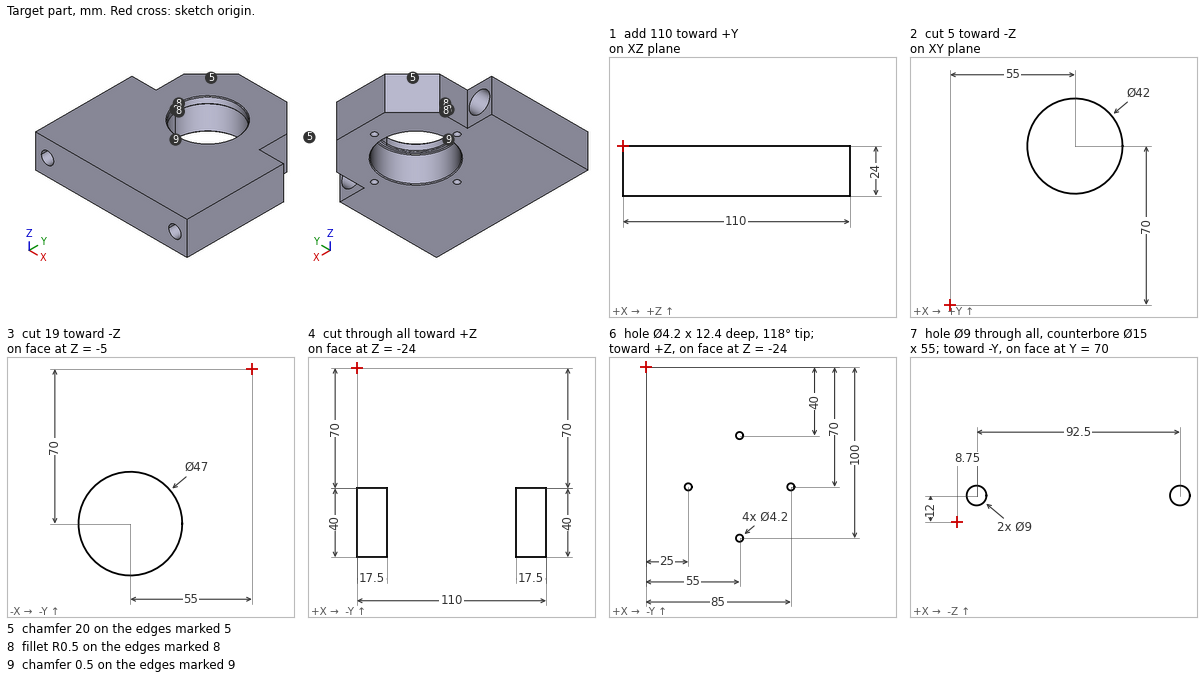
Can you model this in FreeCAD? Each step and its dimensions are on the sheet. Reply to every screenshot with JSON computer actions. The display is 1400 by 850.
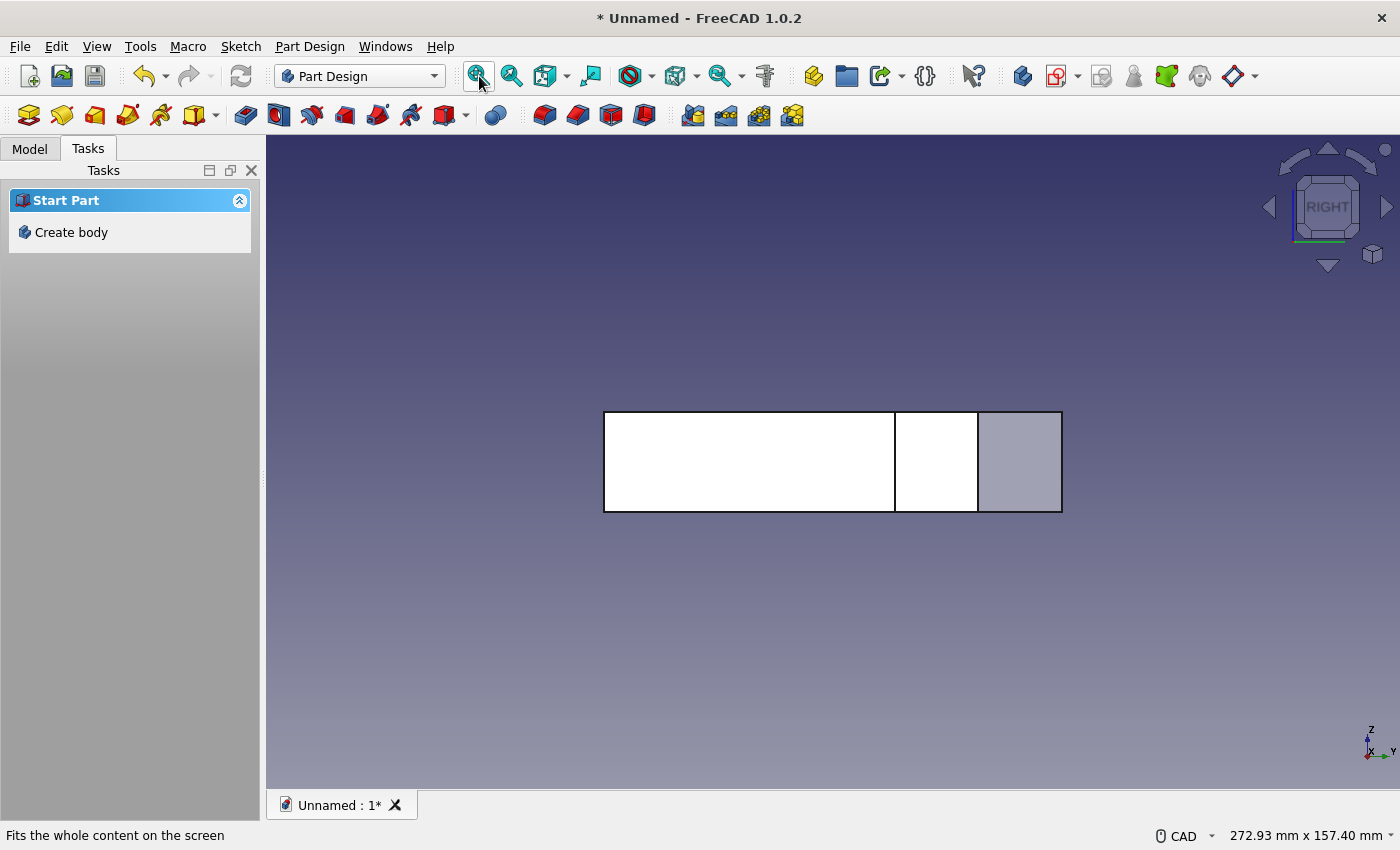
{"action": "left_click", "coordinate": [479, 76]}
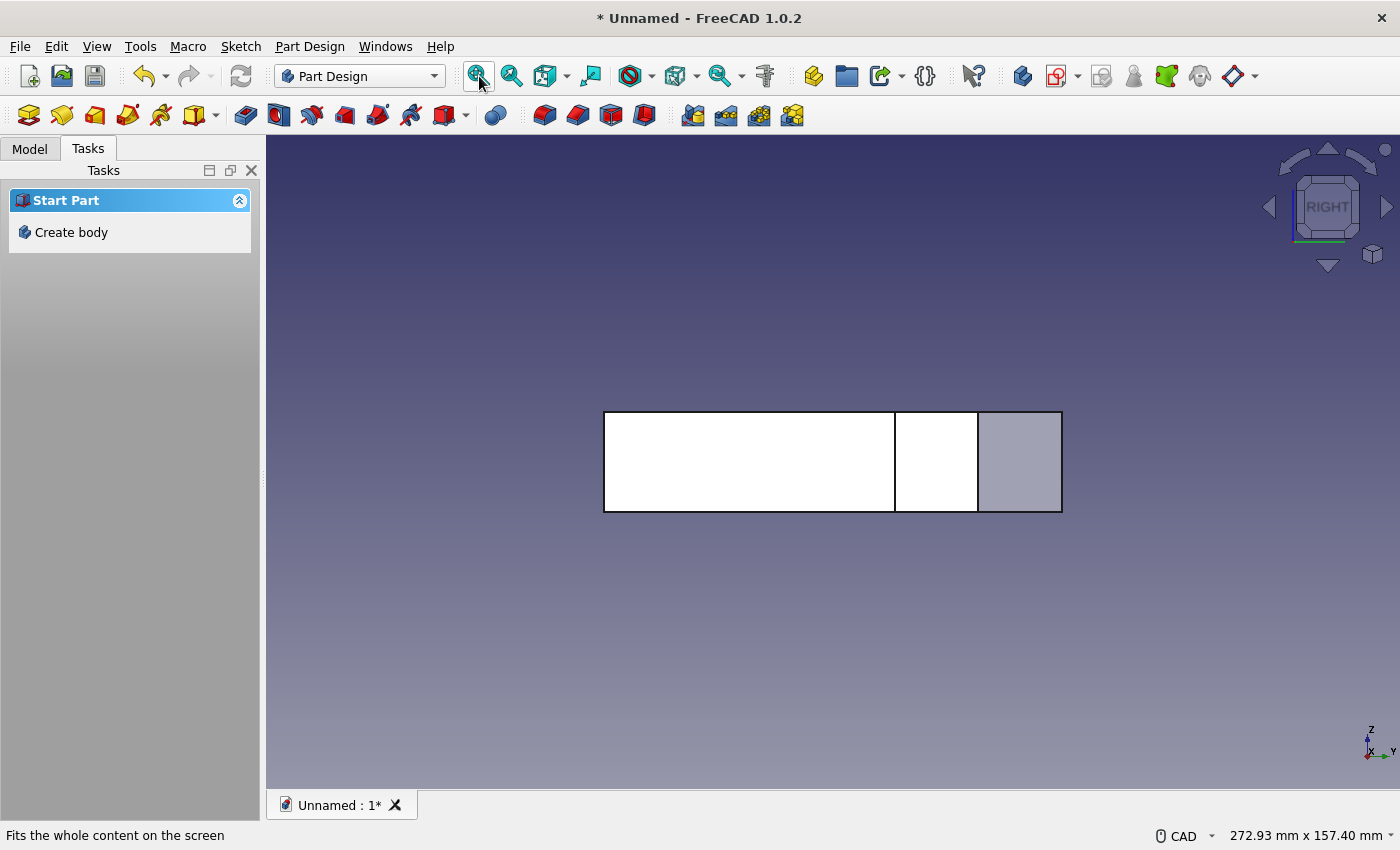
{"action": "key", "text": "5"}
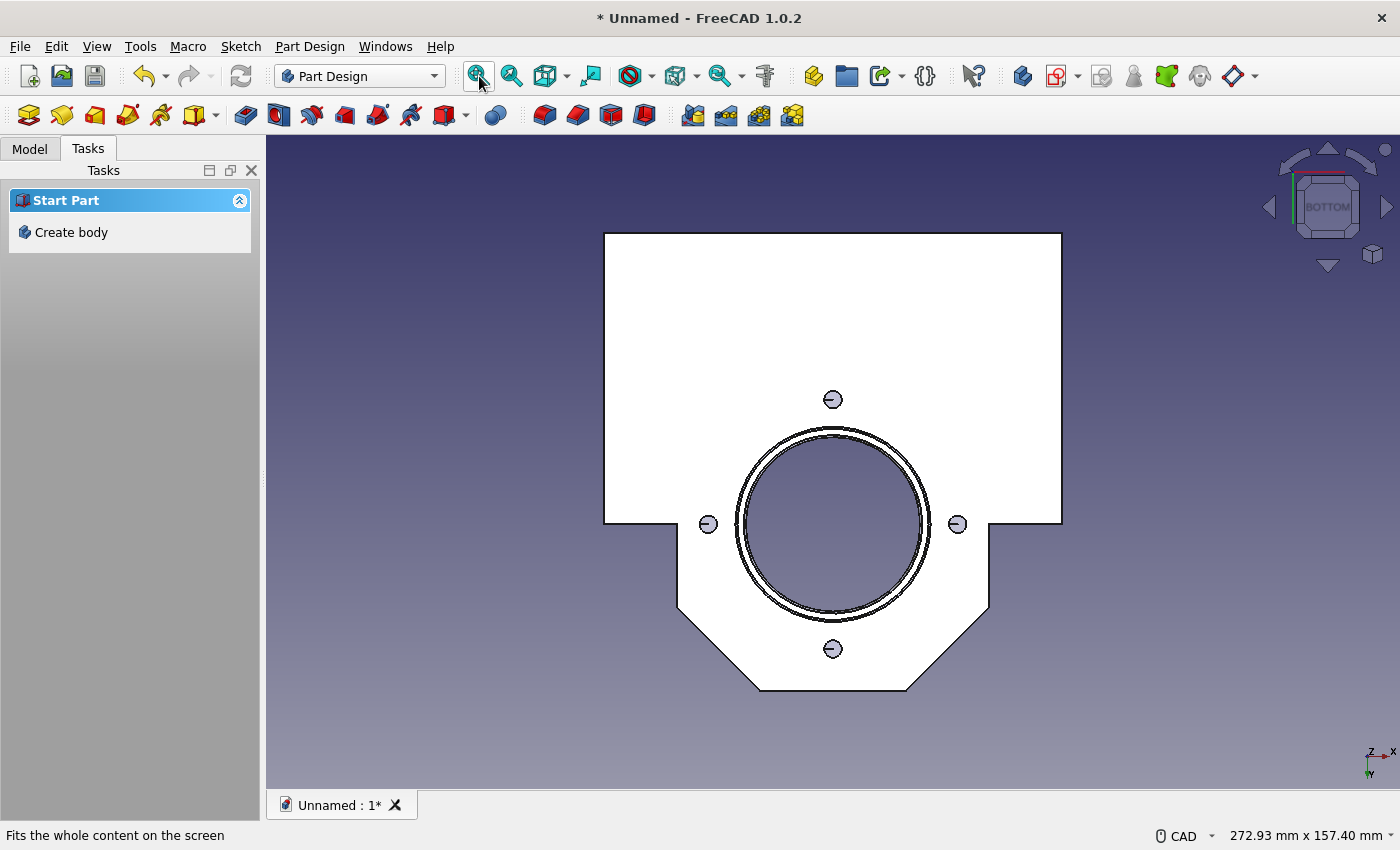
{"action": "left_click", "coordinate": [912, 466]}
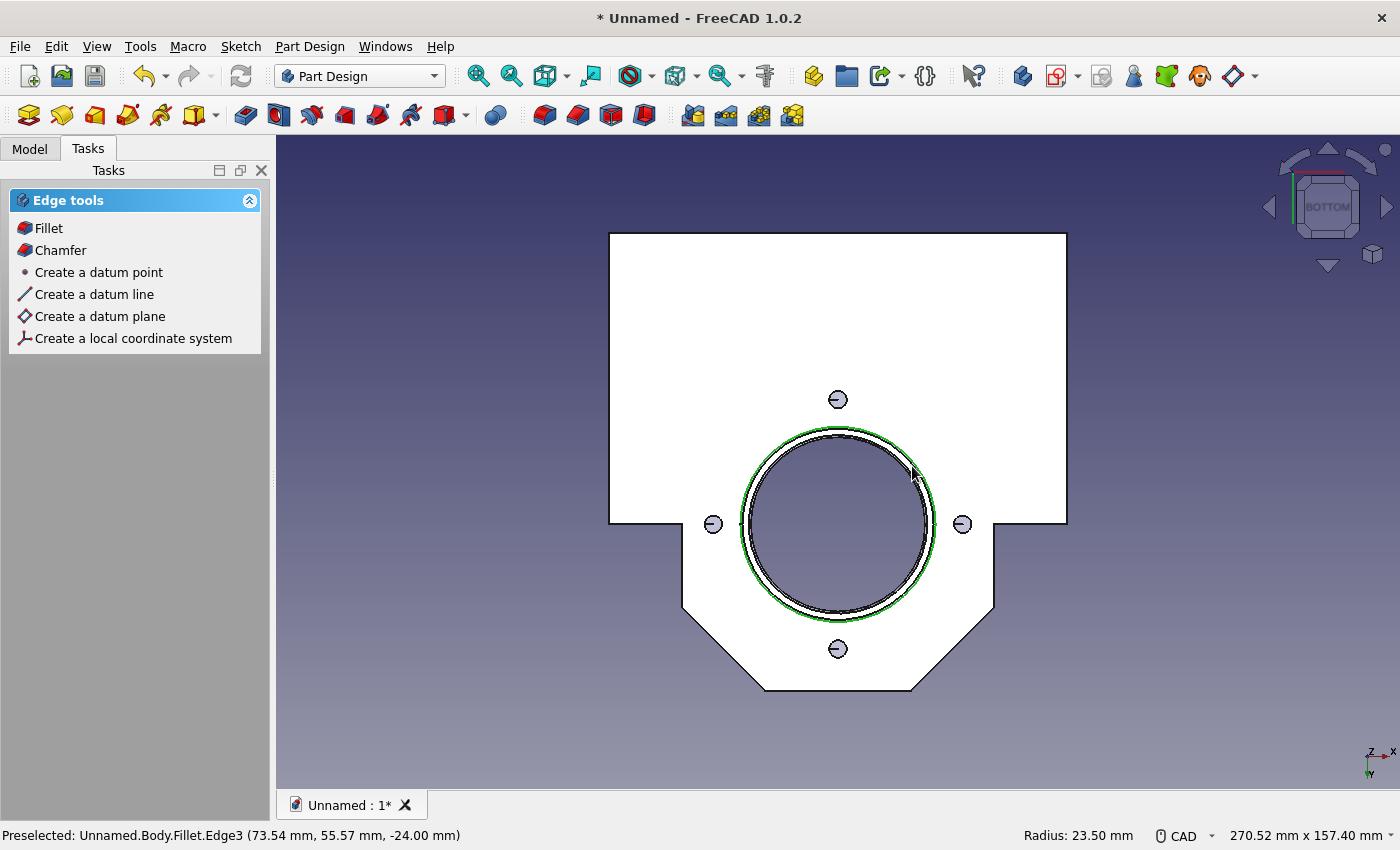
{"action": "left_click", "coordinate": [578, 116]}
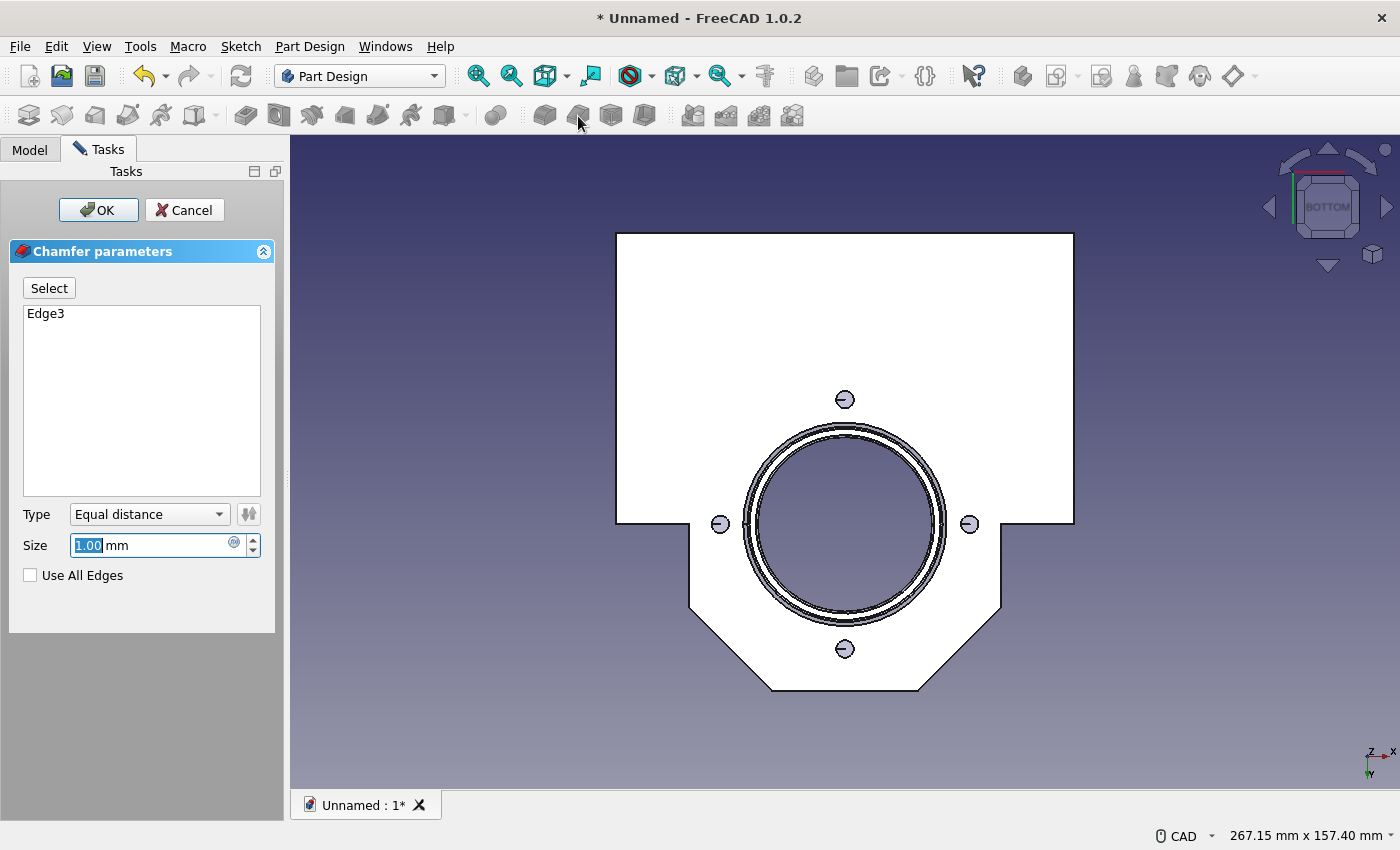
{"action": "type", "text": "0.5"}
{"action": "key", "text": "Tab"}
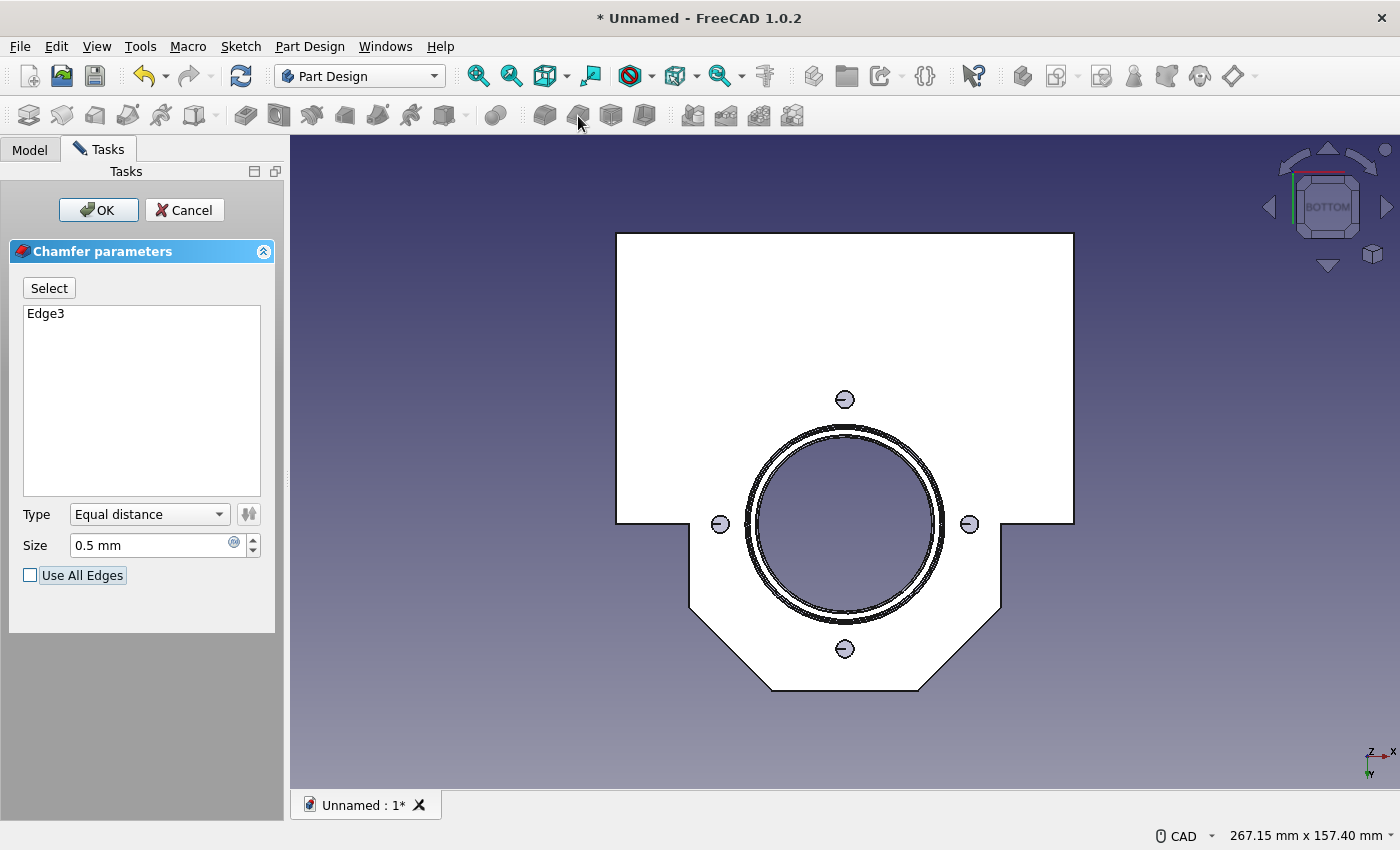
{"action": "left_click", "coordinate": [99, 210]}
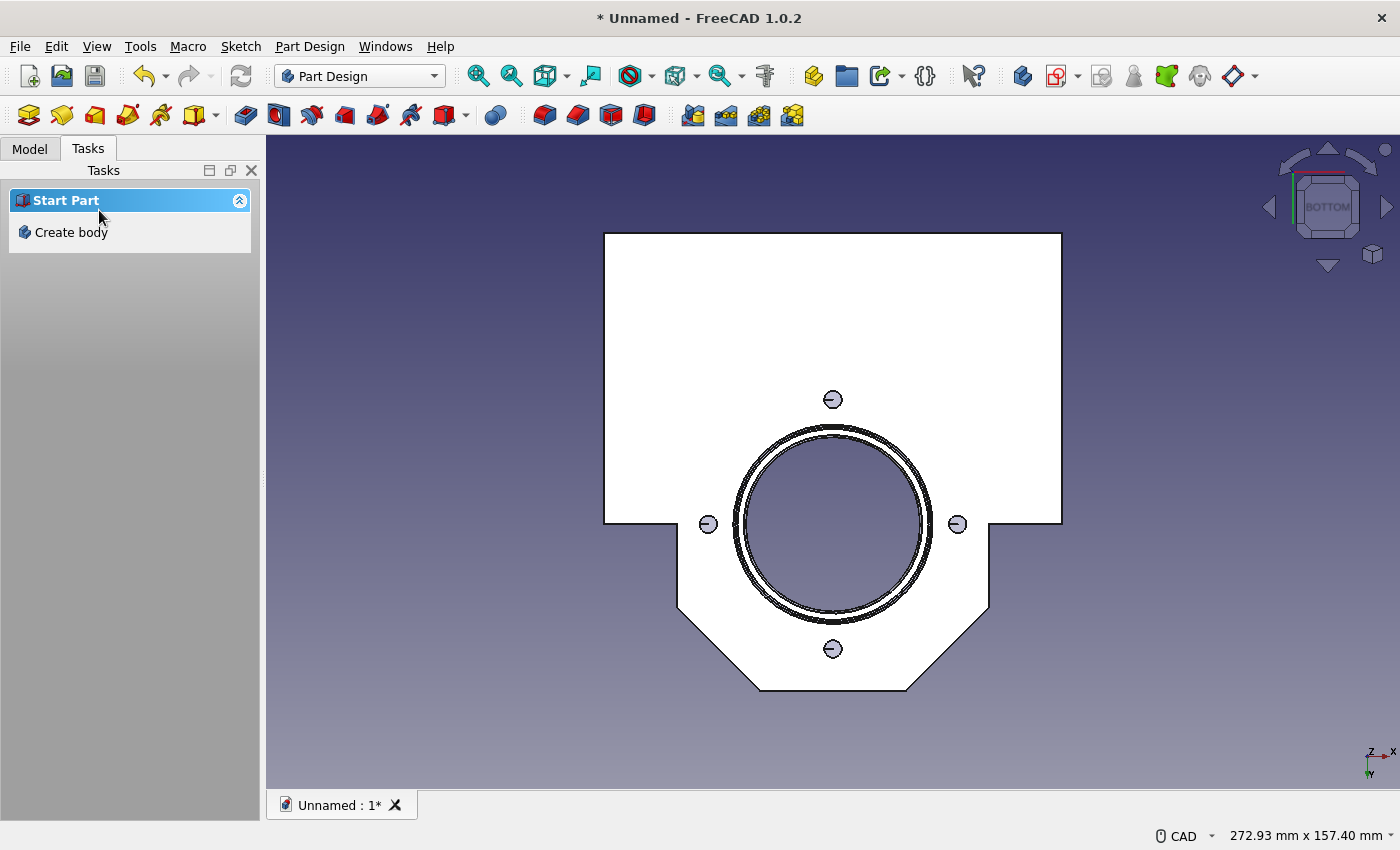
{"action": "key", "text": "0"}